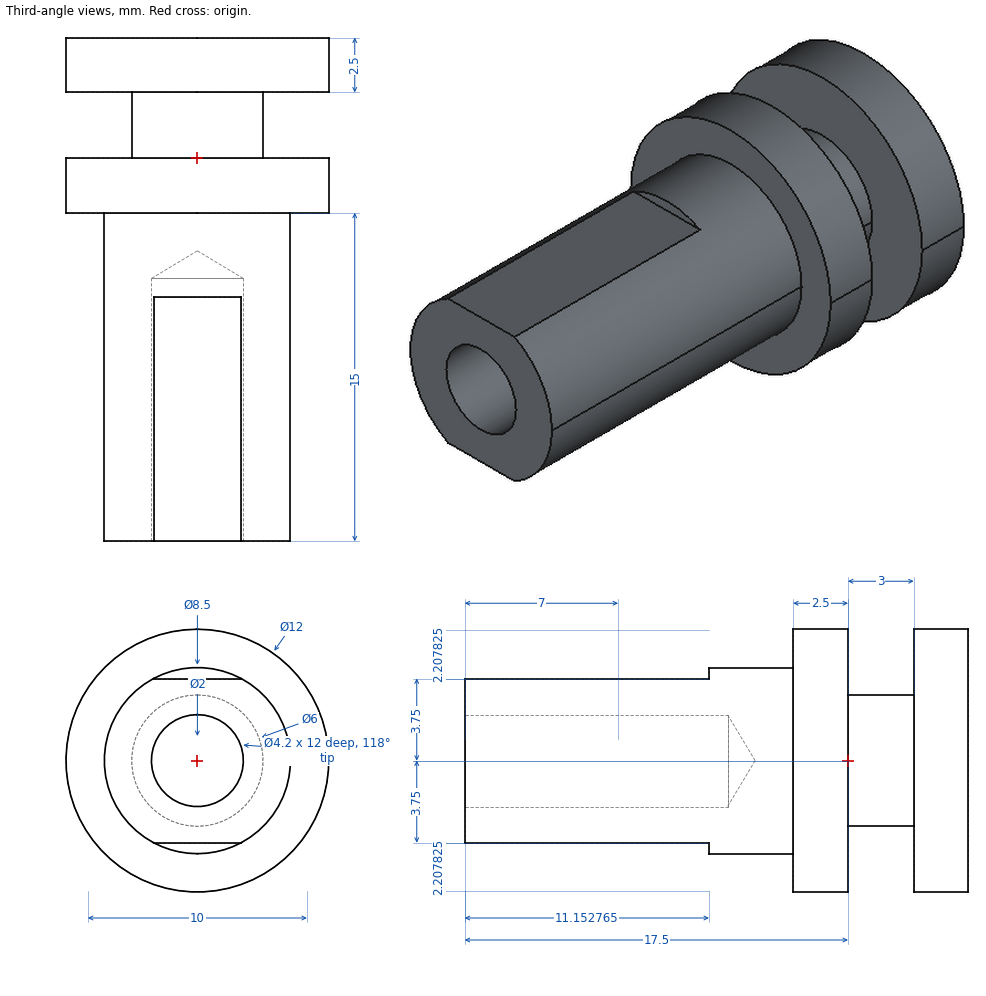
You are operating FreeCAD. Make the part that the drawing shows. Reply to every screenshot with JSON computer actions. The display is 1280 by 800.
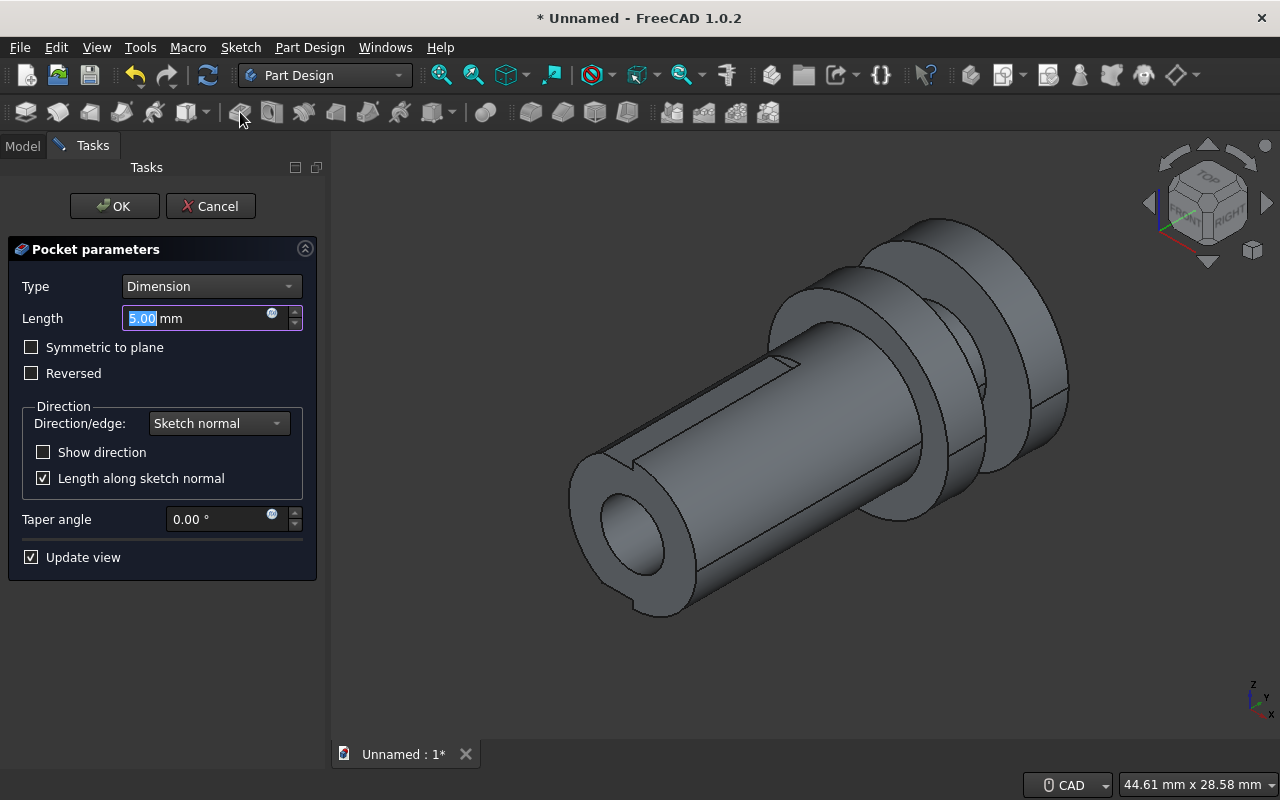
{"action": "type", "text": "10"}
{"action": "key", "text": "Tab"}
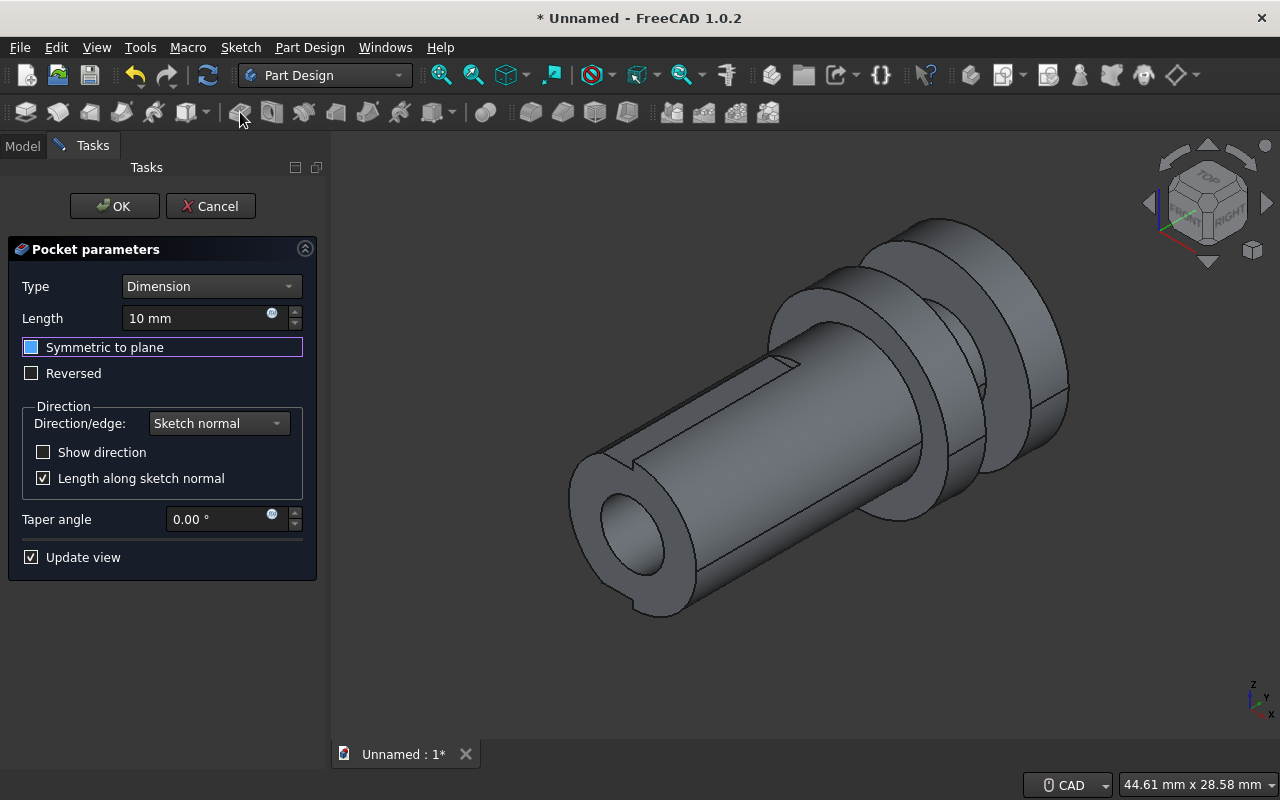
{"action": "left_click", "coordinate": [30, 347]}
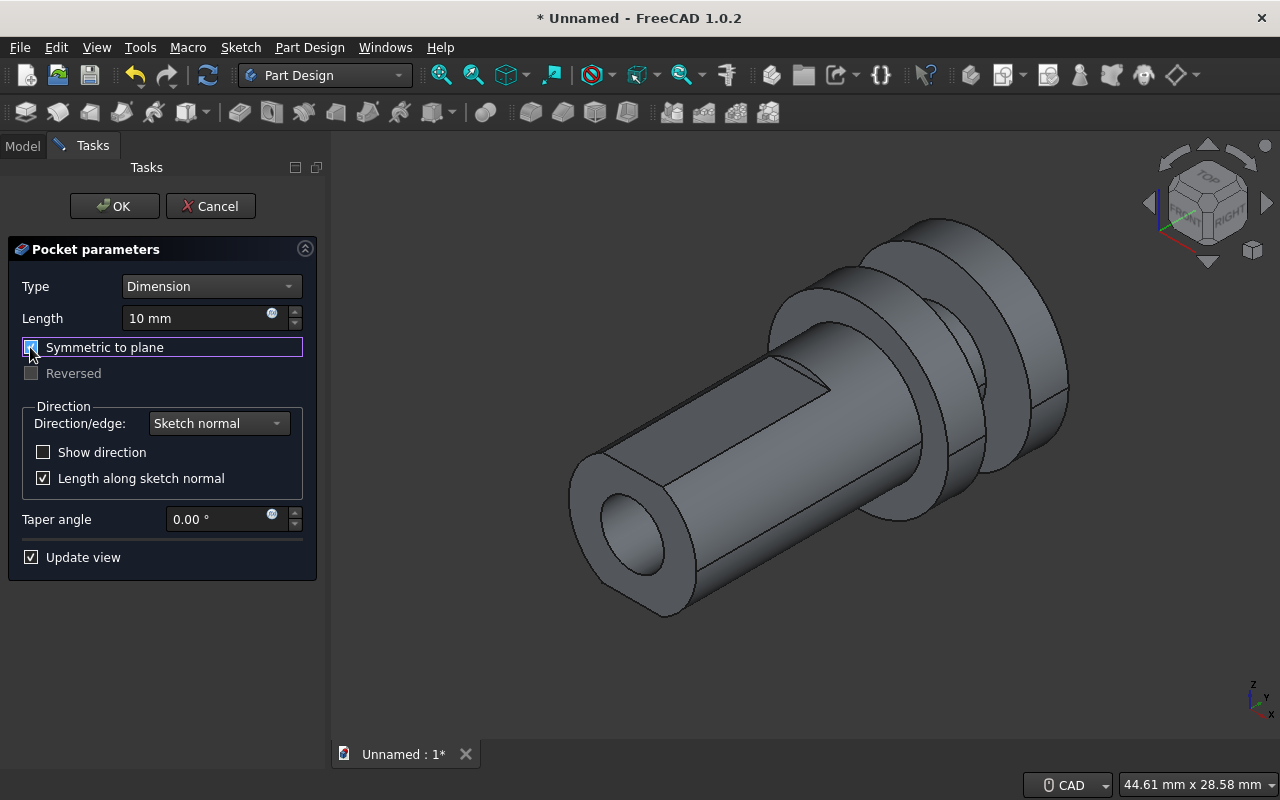
{"action": "left_click", "coordinate": [115, 206]}